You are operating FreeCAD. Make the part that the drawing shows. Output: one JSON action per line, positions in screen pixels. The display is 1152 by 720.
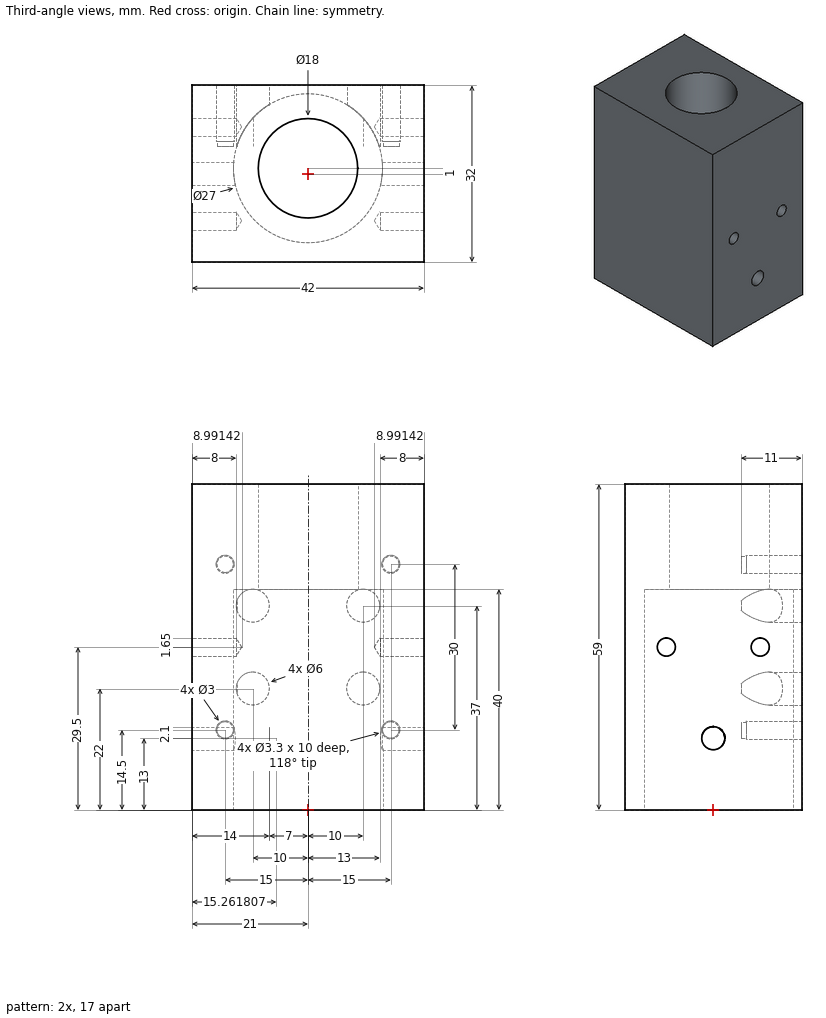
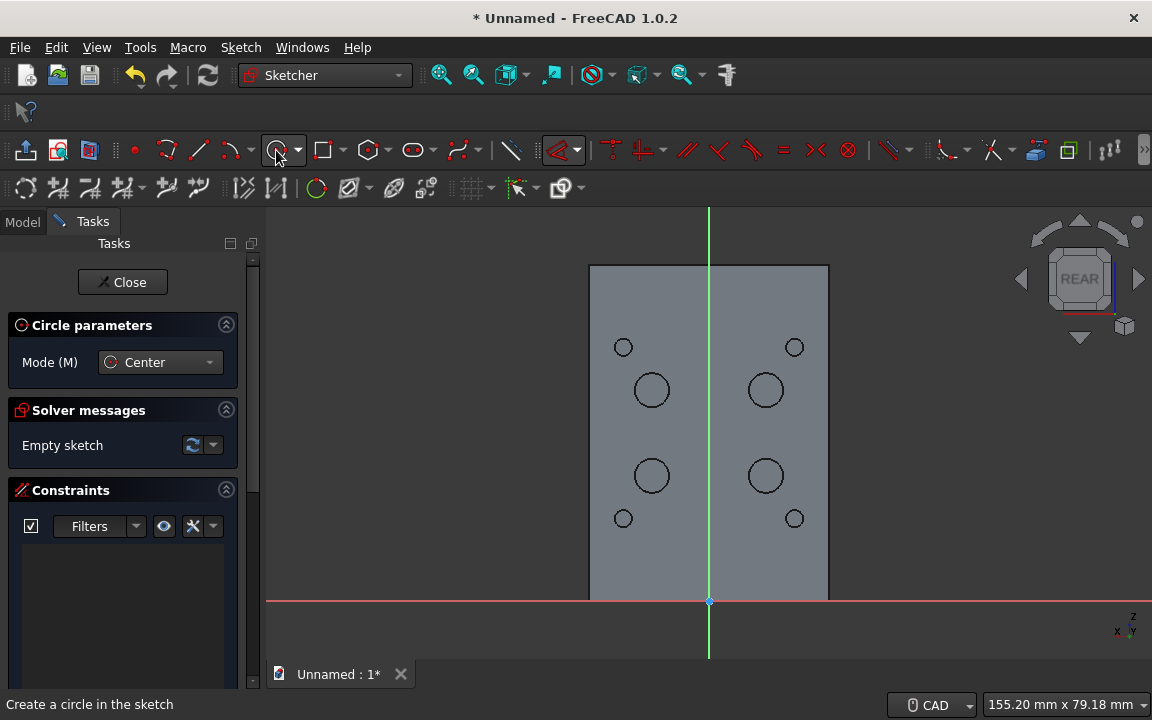
{"action": "scroll", "coordinate": [623, 519], "scroll_direction": "up", "scroll_amount": 5}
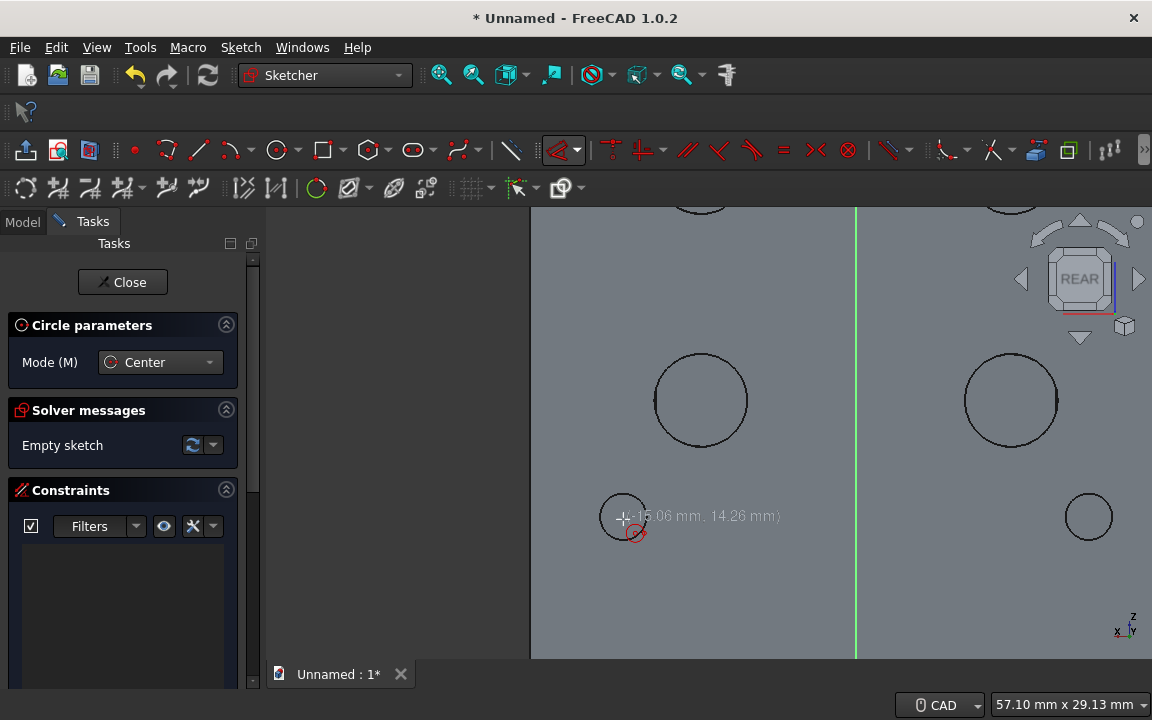
{"action": "left_click", "coordinate": [623, 517]}
{"action": "left_click", "coordinate": [641, 499]}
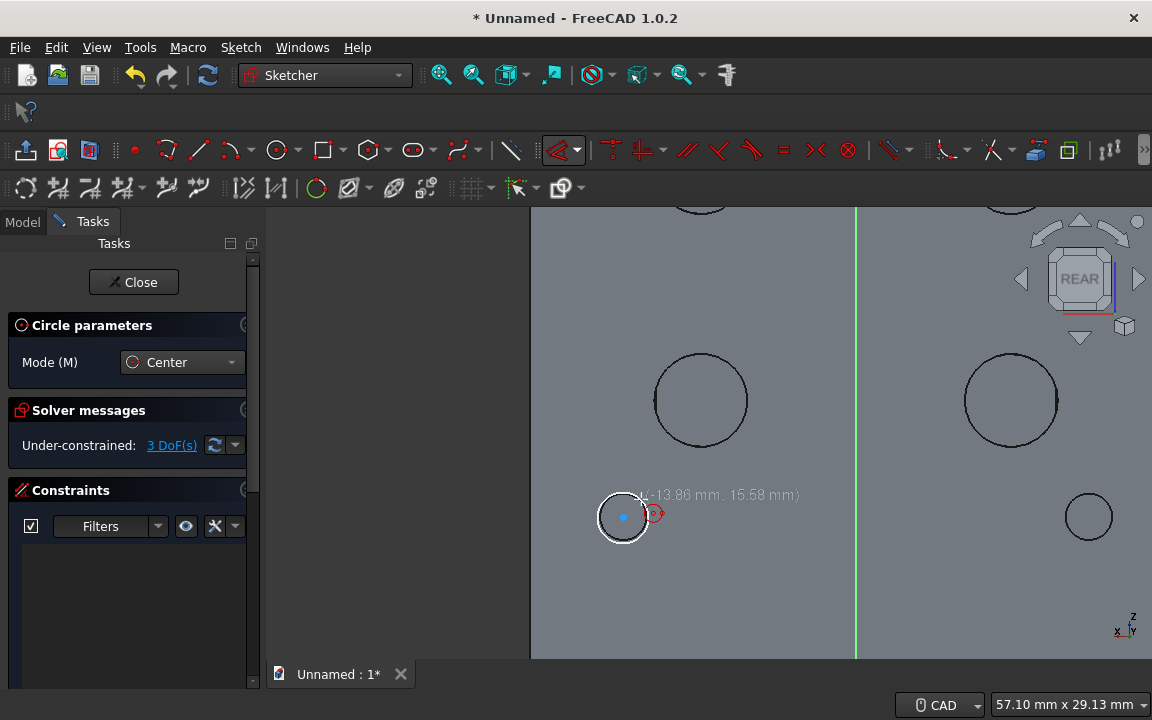
{"action": "scroll", "coordinate": [515, 462], "scroll_direction": "down", "scroll_amount": 5}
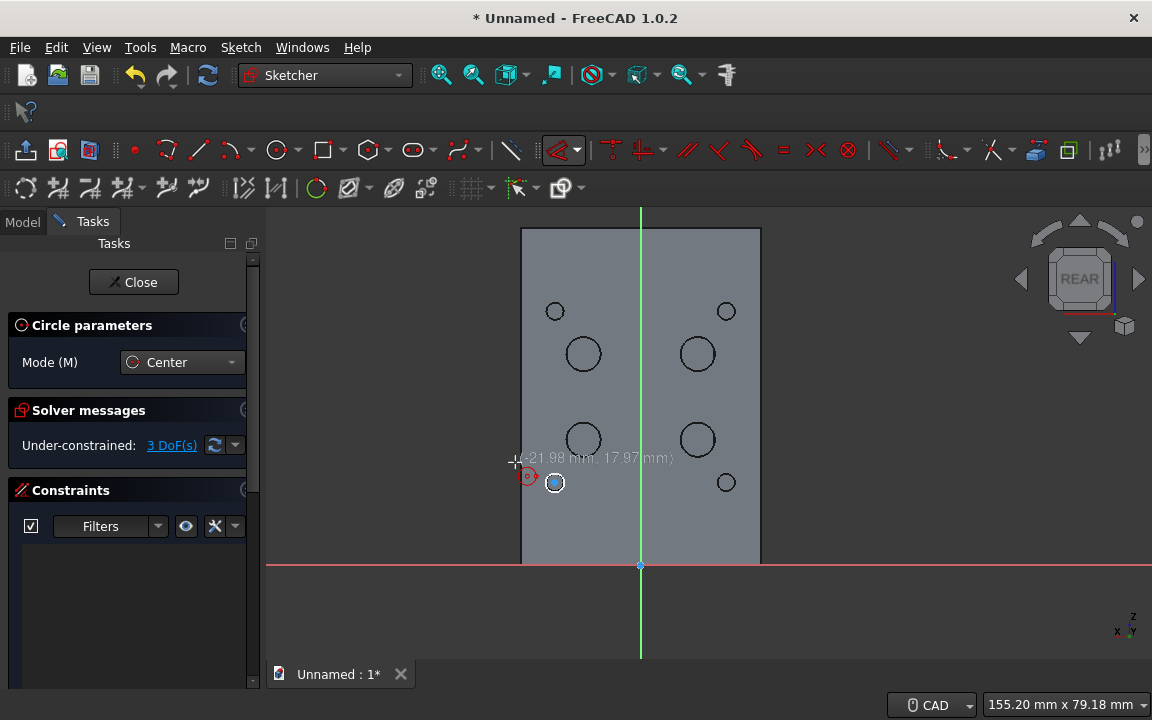
{"action": "scroll", "coordinate": [555, 311], "scroll_direction": "up", "scroll_amount": 5}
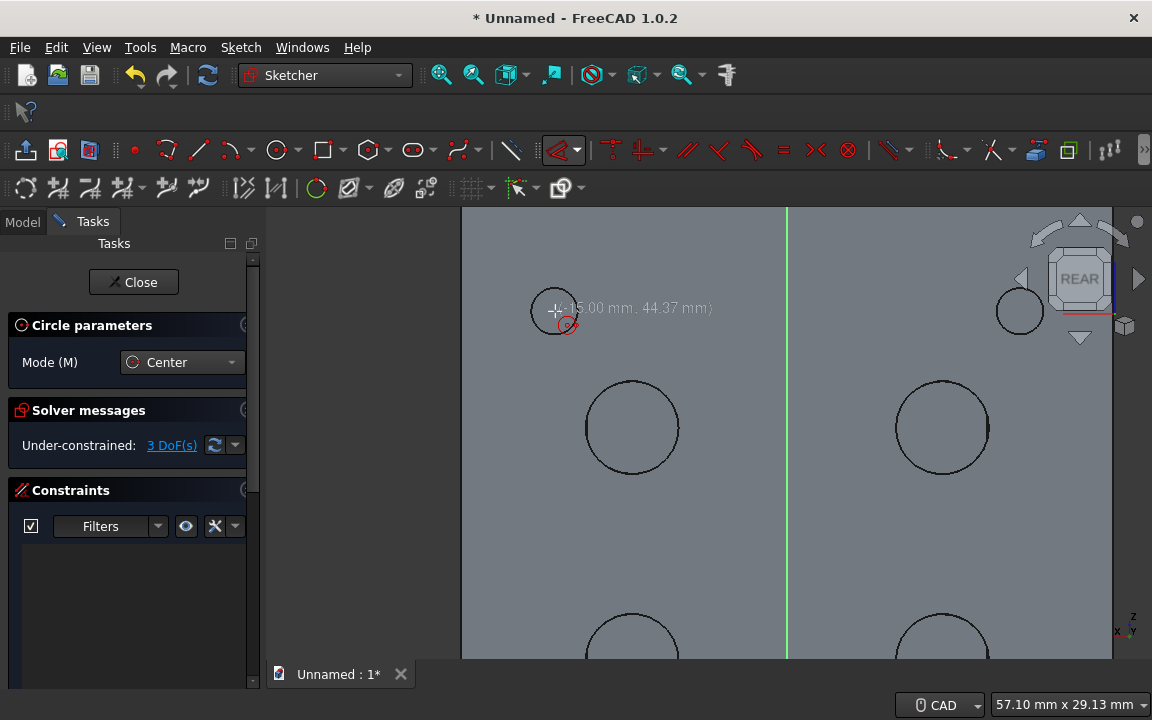
{"action": "left_click", "coordinate": [555, 311]}
{"action": "left_click", "coordinate": [573, 293]}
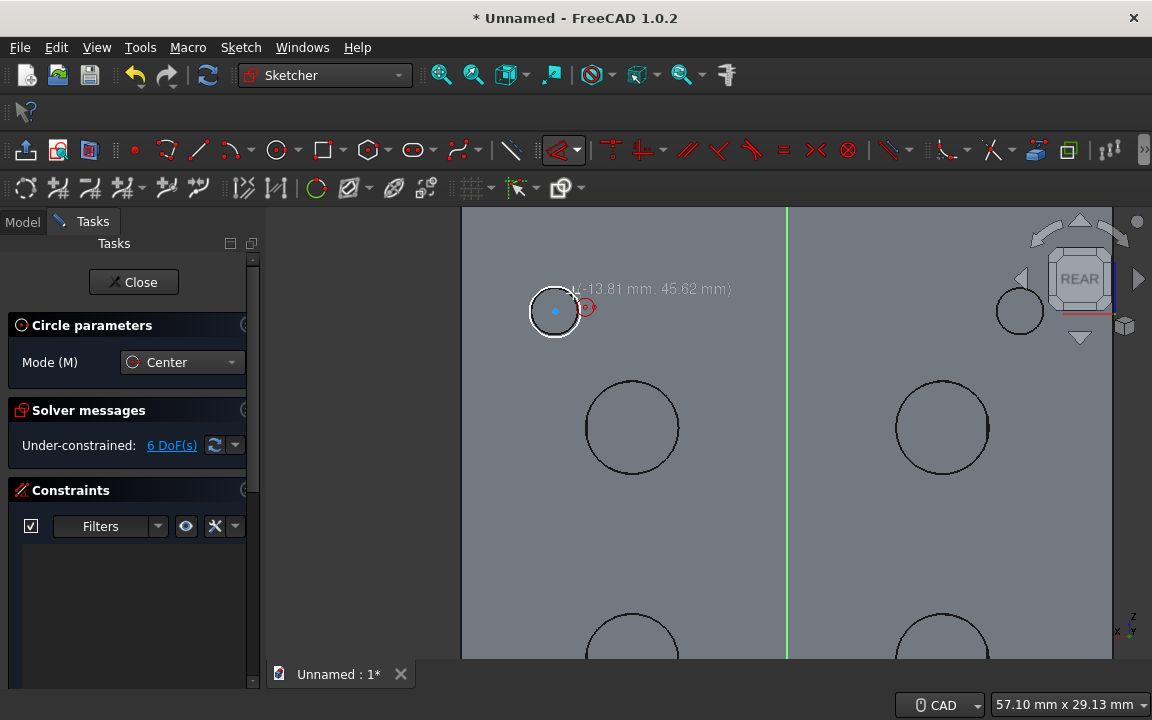
{"action": "scroll", "coordinate": [555, 310], "scroll_direction": "down", "scroll_amount": 5}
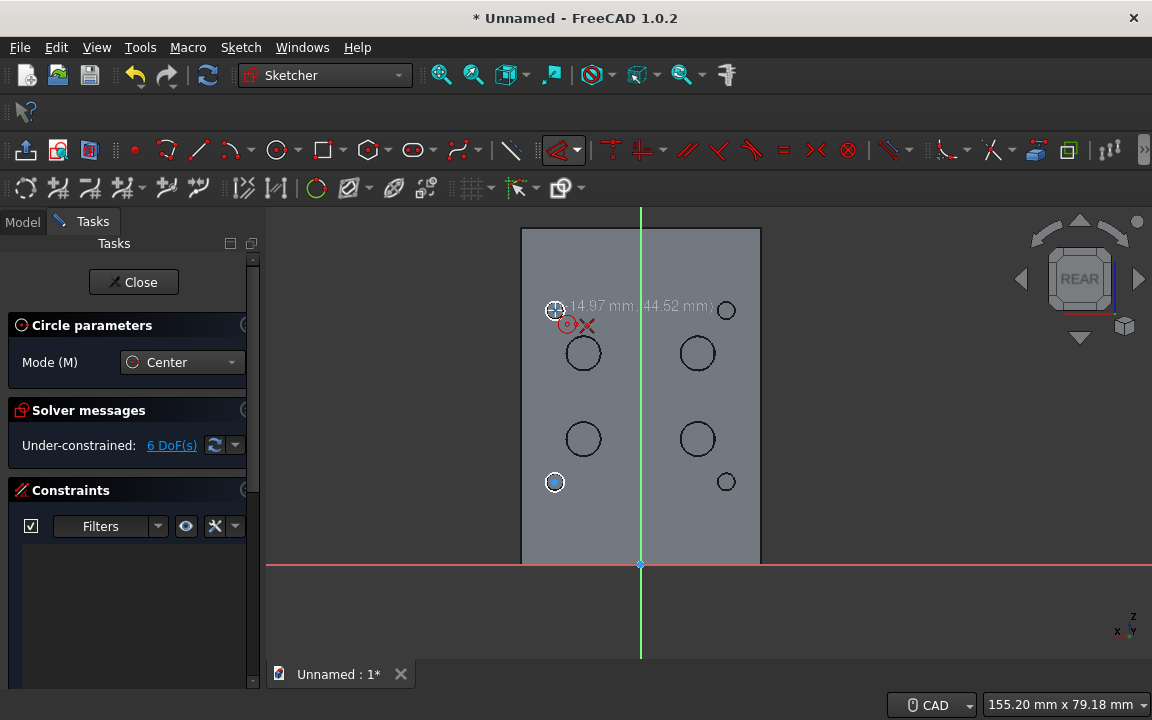
{"action": "scroll", "coordinate": [726, 311], "scroll_direction": "up", "scroll_amount": 5}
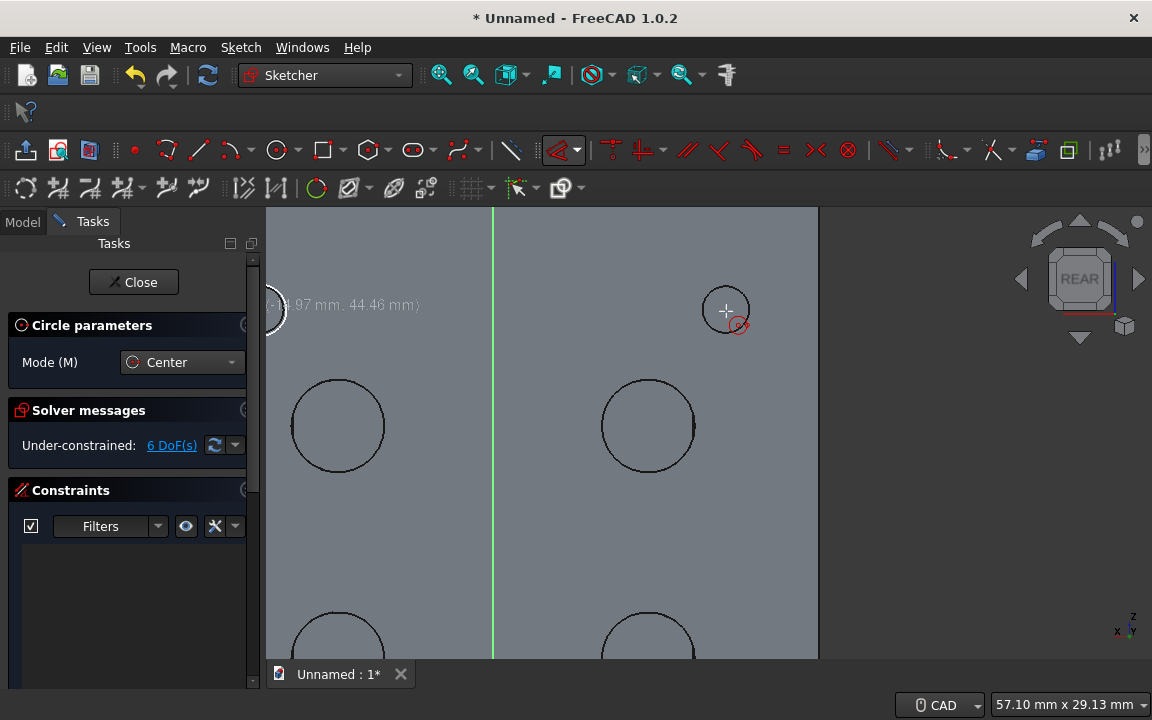
{"action": "left_click", "coordinate": [726, 310]}
{"action": "left_click", "coordinate": [744, 291]}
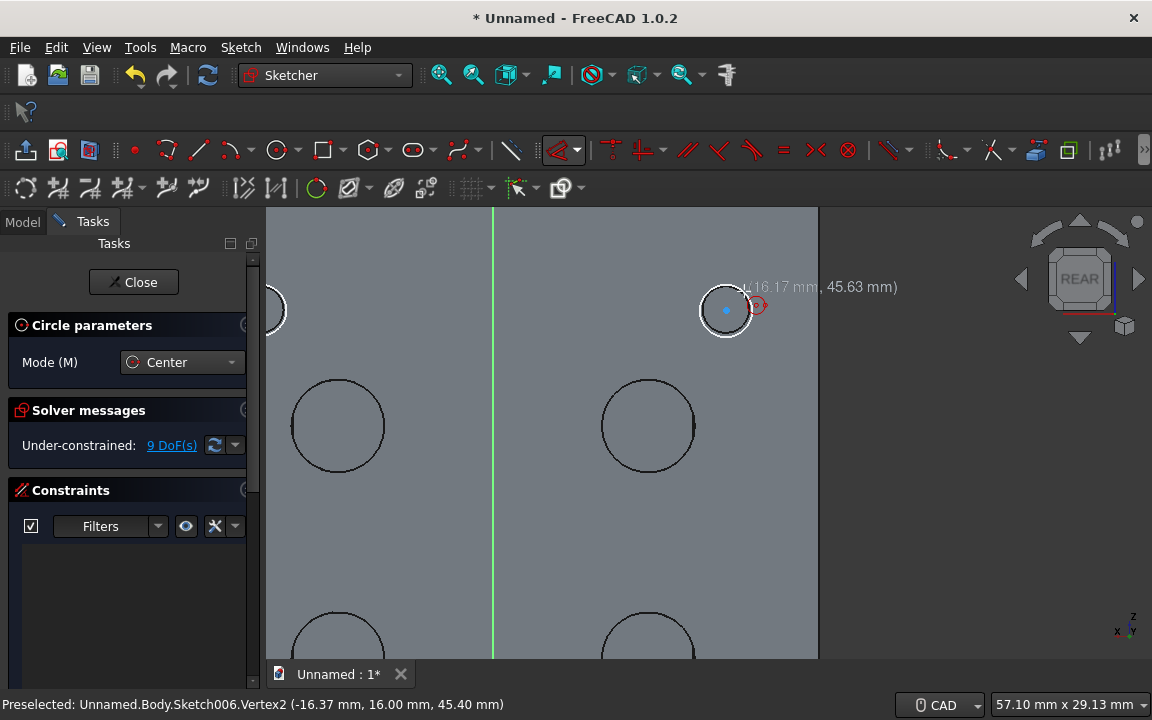
{"action": "scroll", "coordinate": [726, 311], "scroll_direction": "down", "scroll_amount": 5}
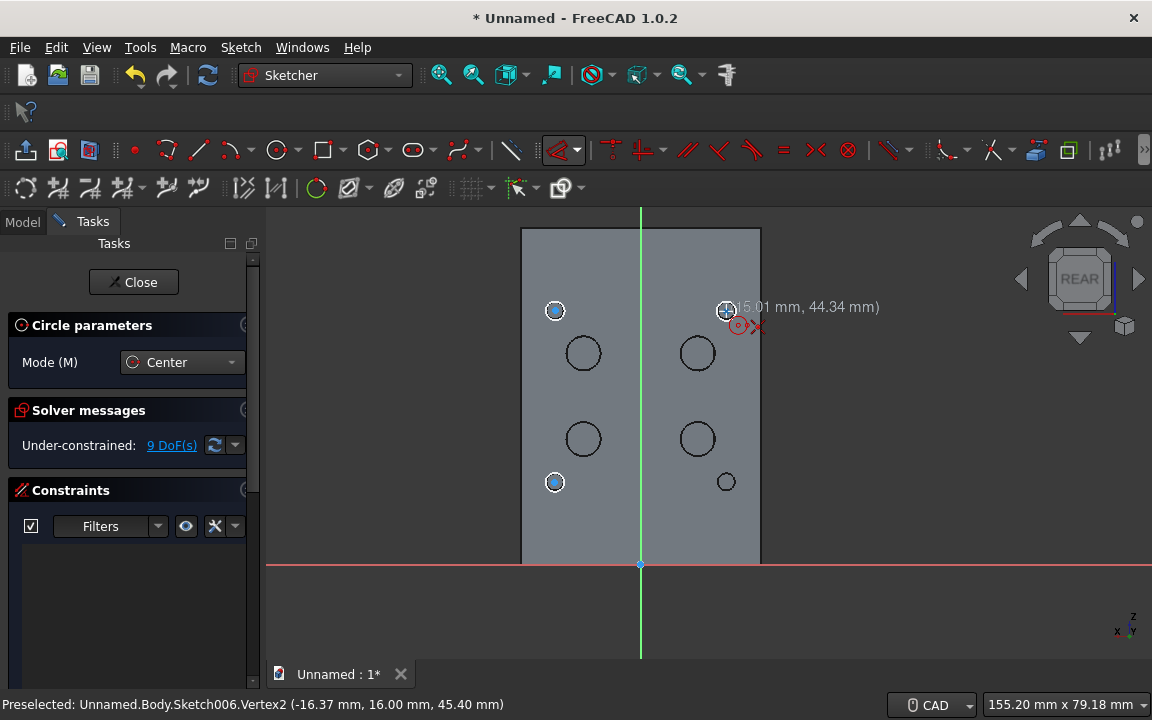
{"action": "scroll", "coordinate": [726, 482], "scroll_direction": "up", "scroll_amount": 5}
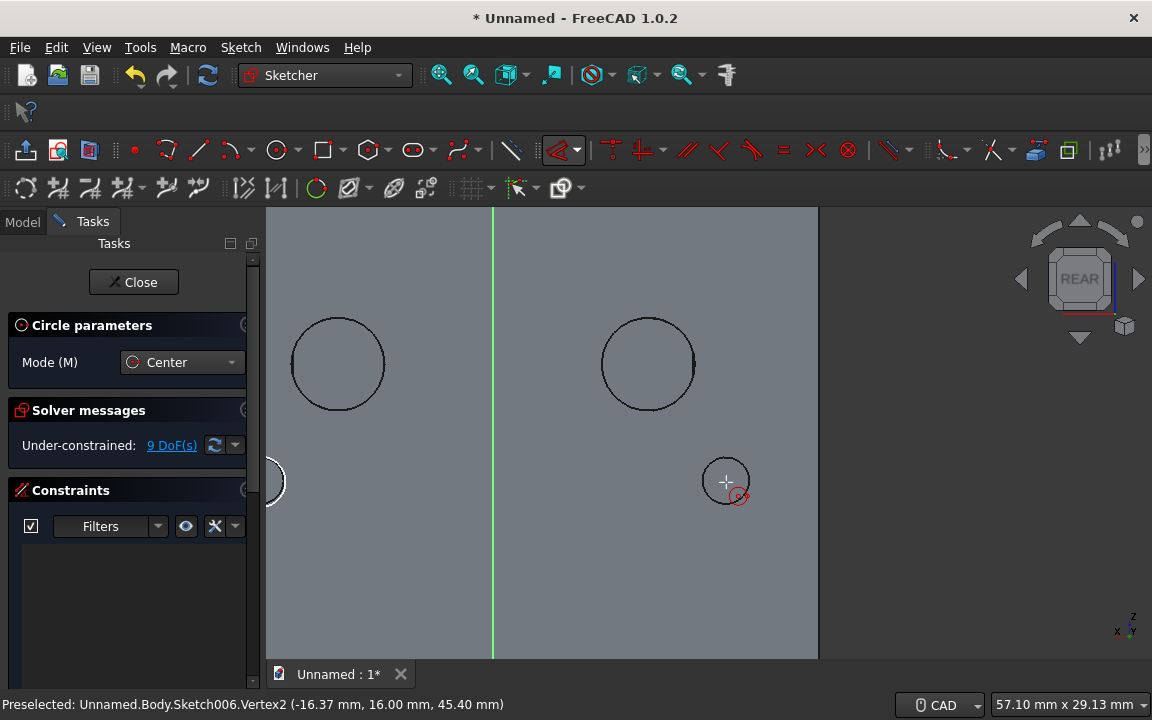
{"action": "left_click", "coordinate": [726, 481]}
{"action": "left_click", "coordinate": [744, 463]}
{"action": "key", "text": "Escape"}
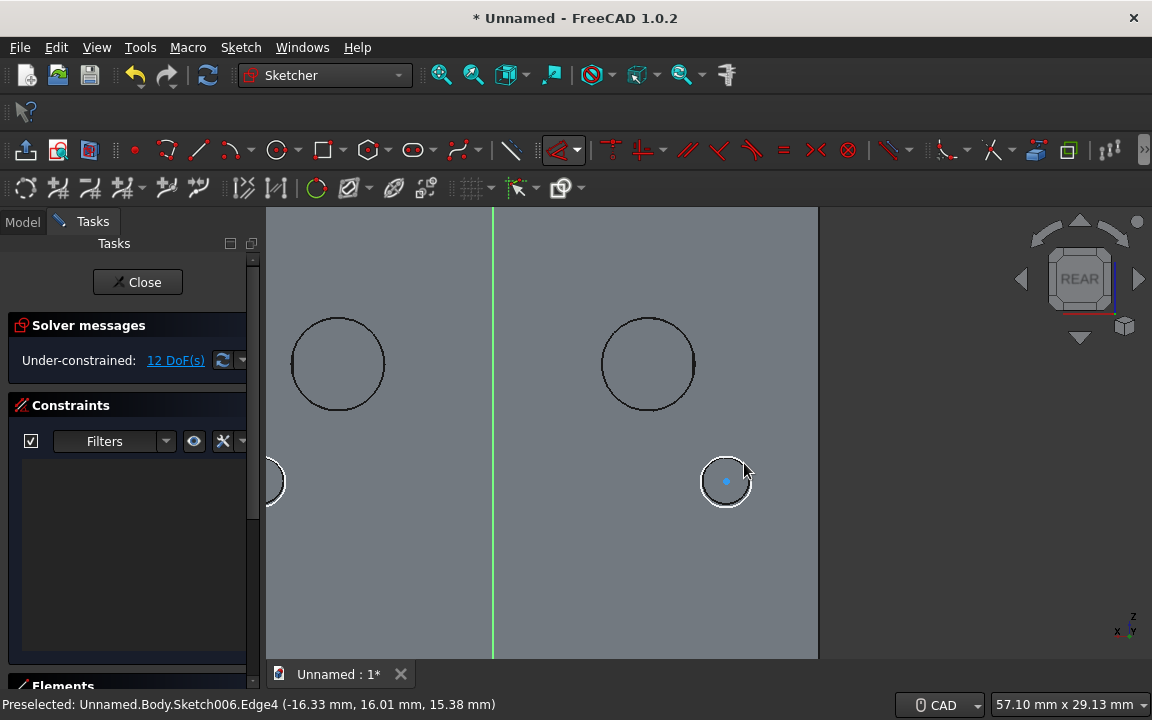
{"action": "scroll", "coordinate": [726, 483], "scroll_direction": "down", "scroll_amount": 5}